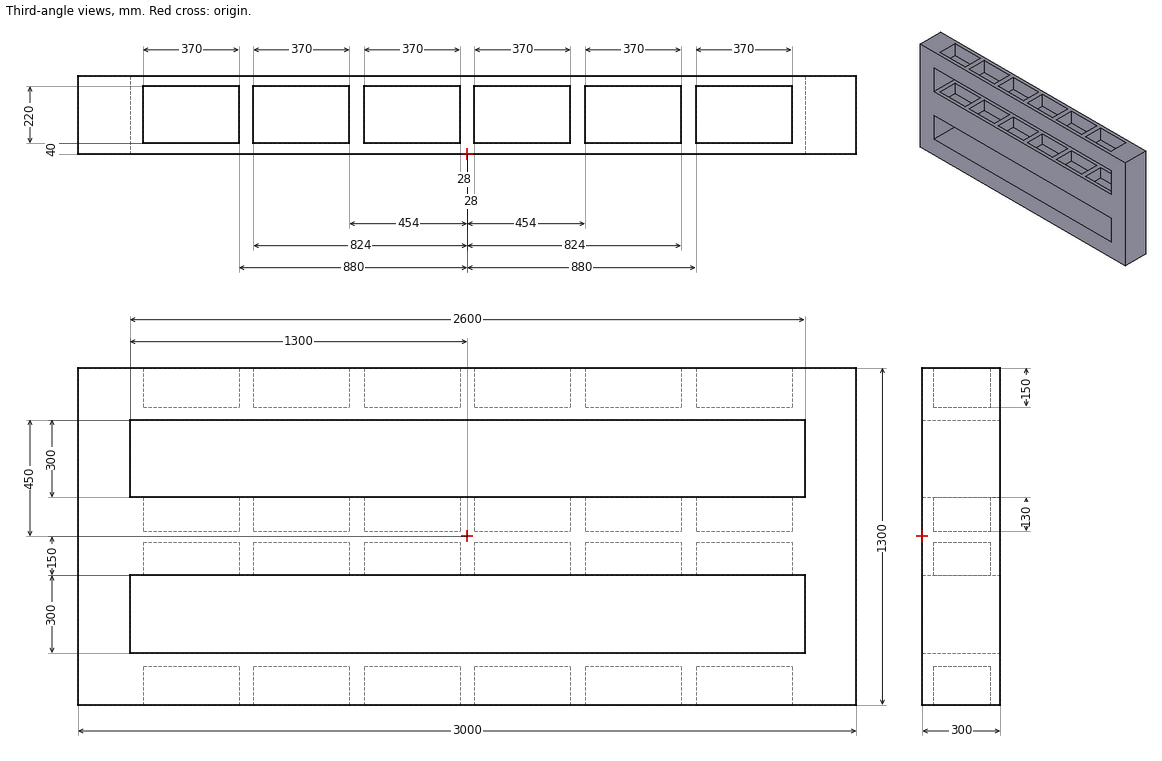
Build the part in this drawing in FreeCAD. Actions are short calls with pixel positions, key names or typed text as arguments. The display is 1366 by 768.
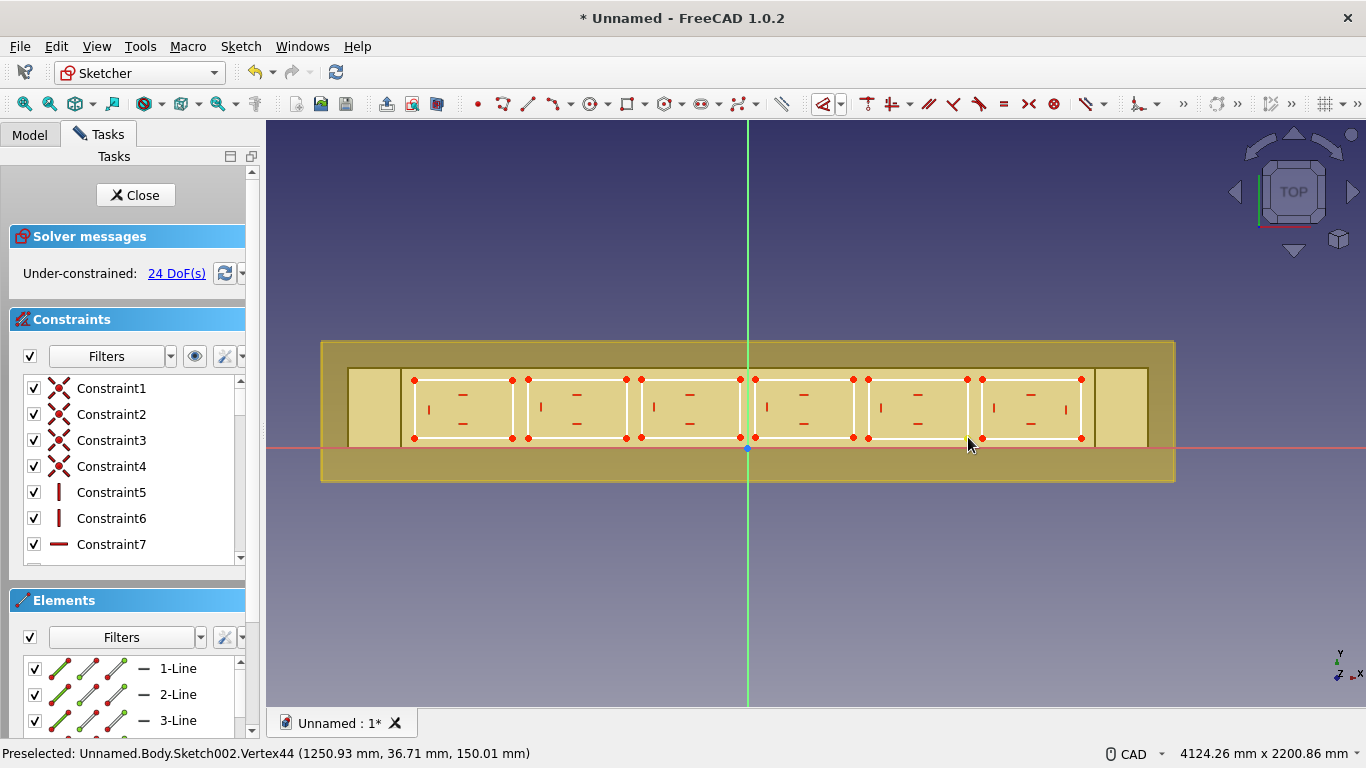
click(415, 398)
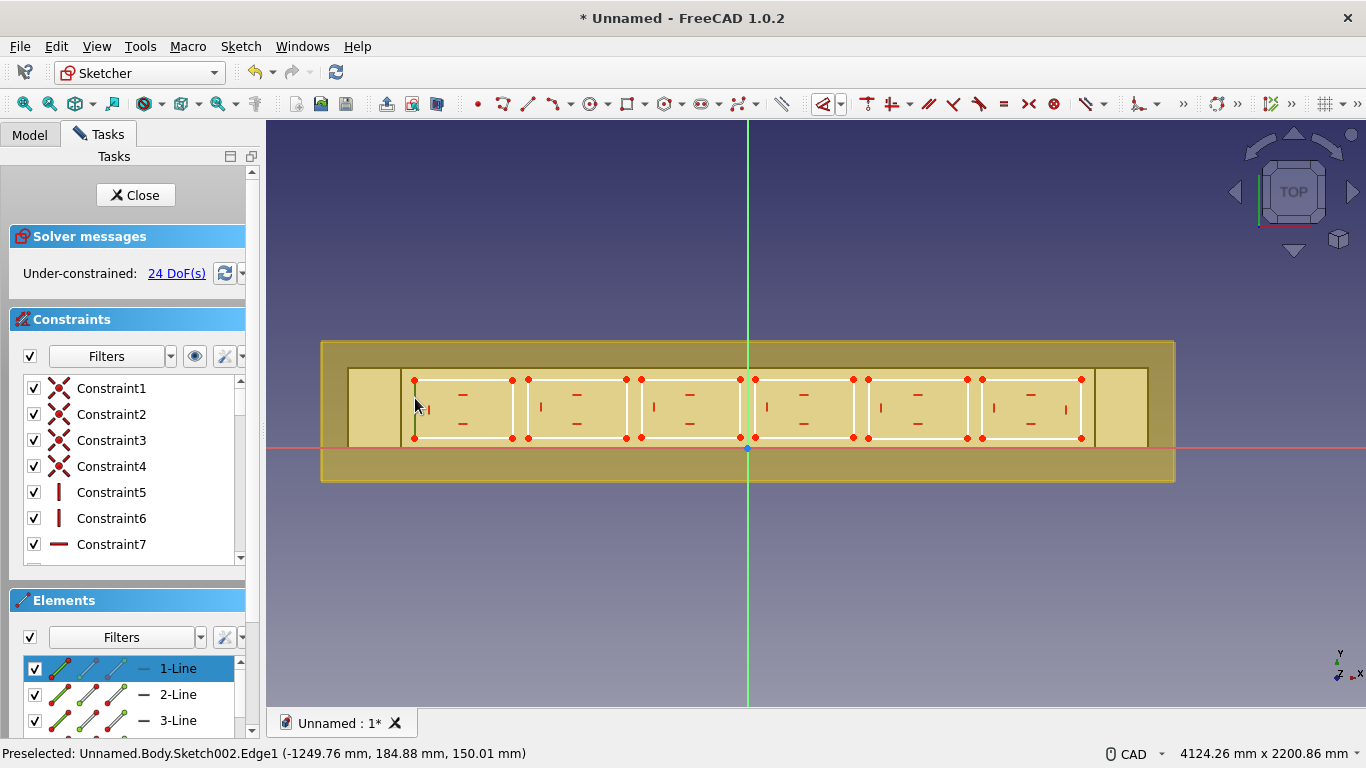
key(i)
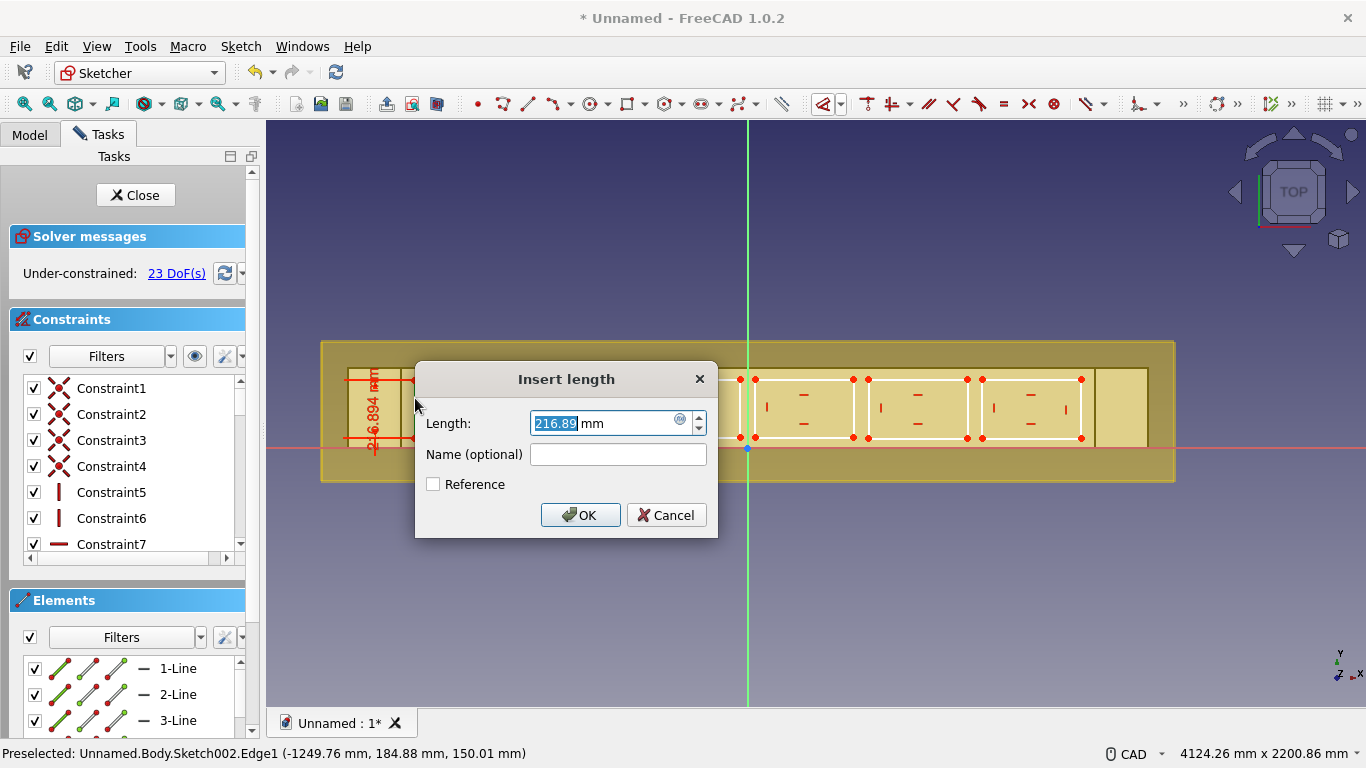
text(220)
key(Return)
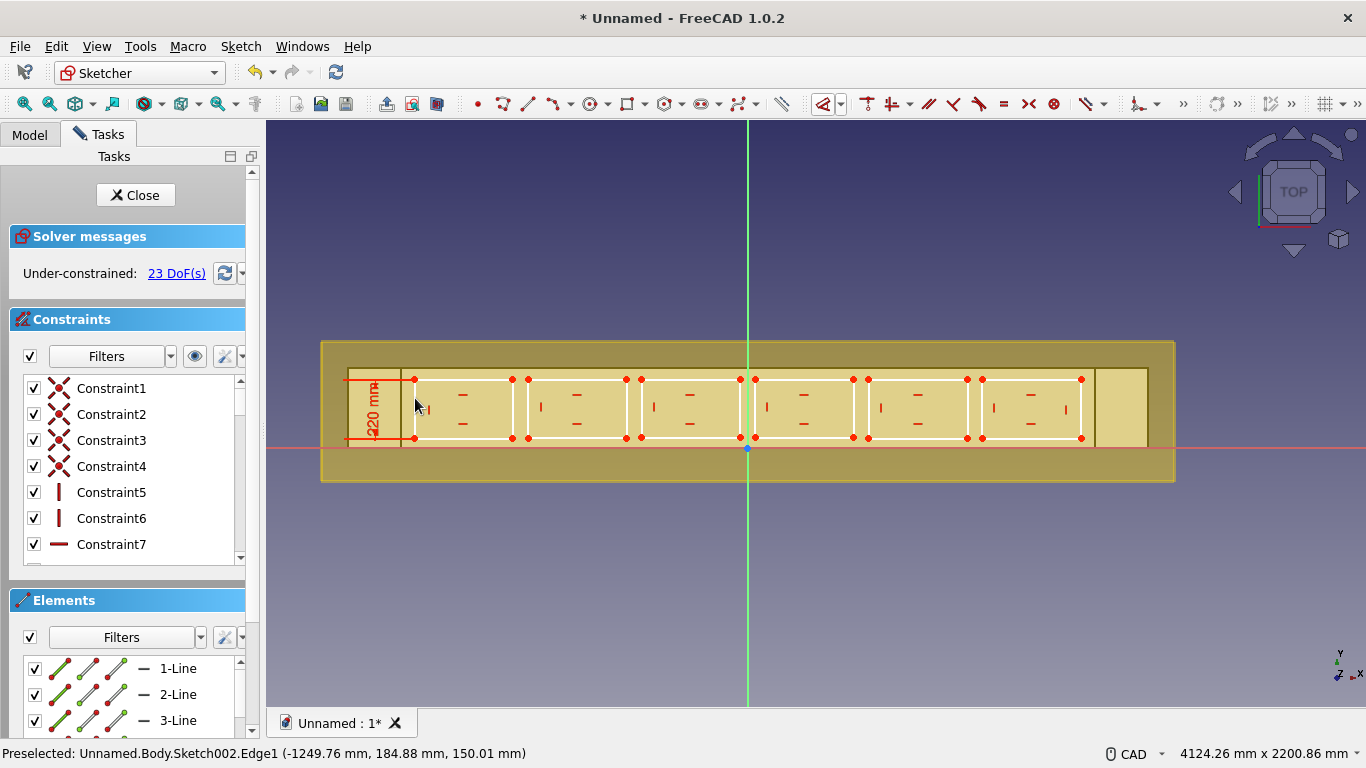
scroll(444, 439, up, 2)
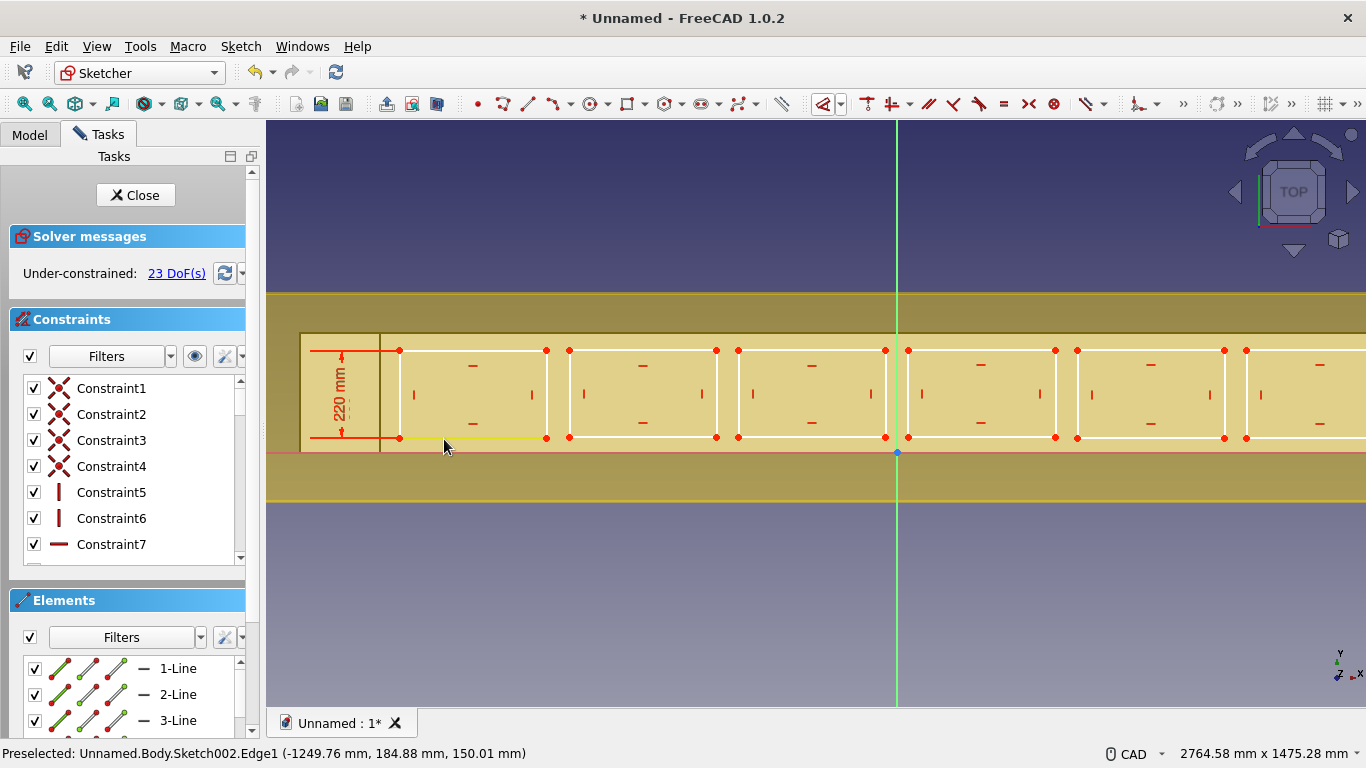
click(444, 438)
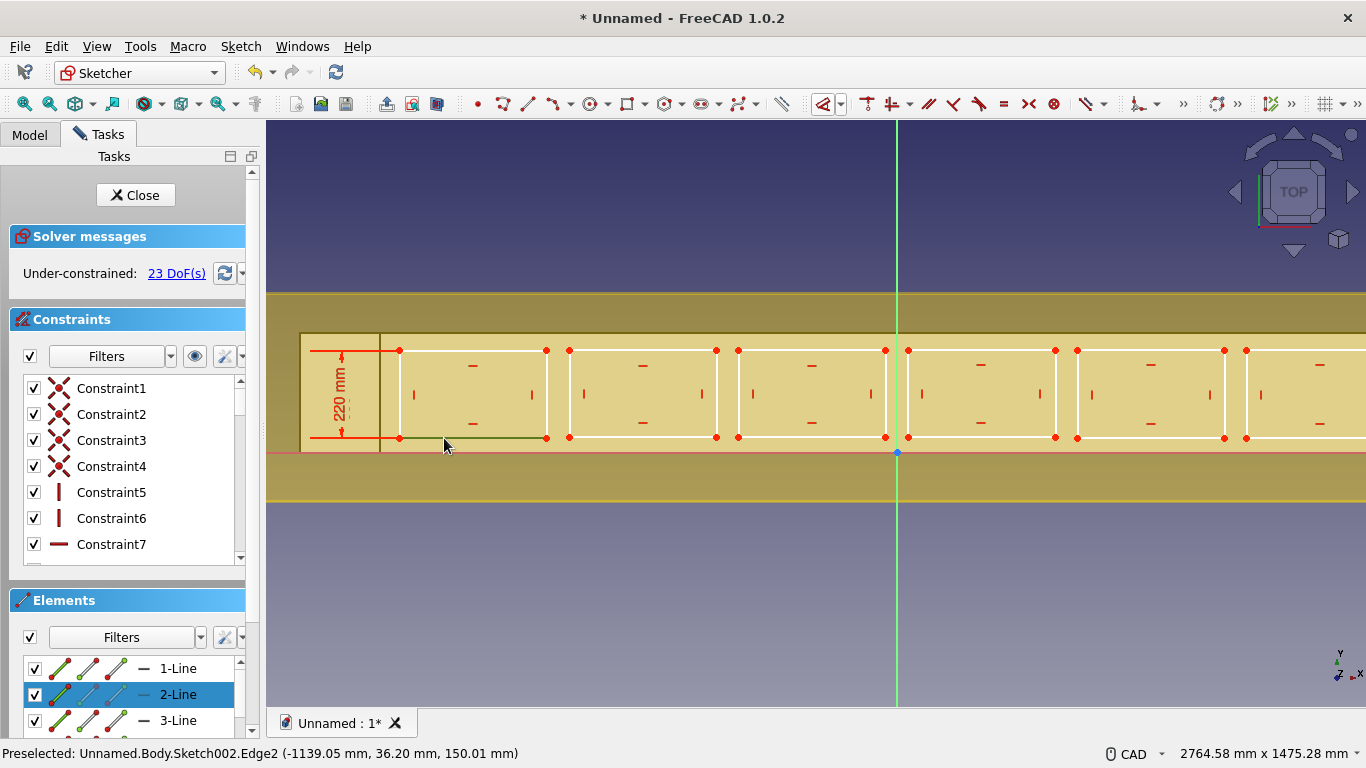
key(l)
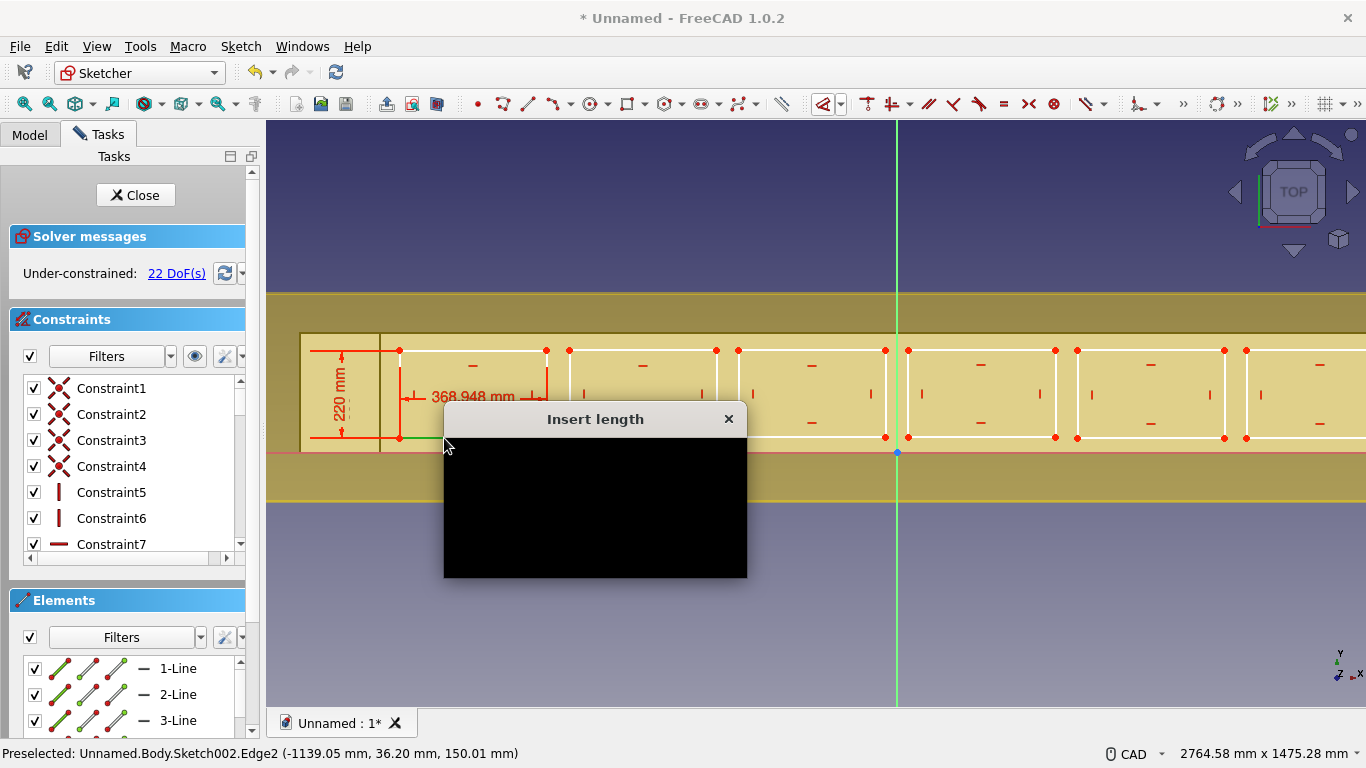
text(370)
key(Return)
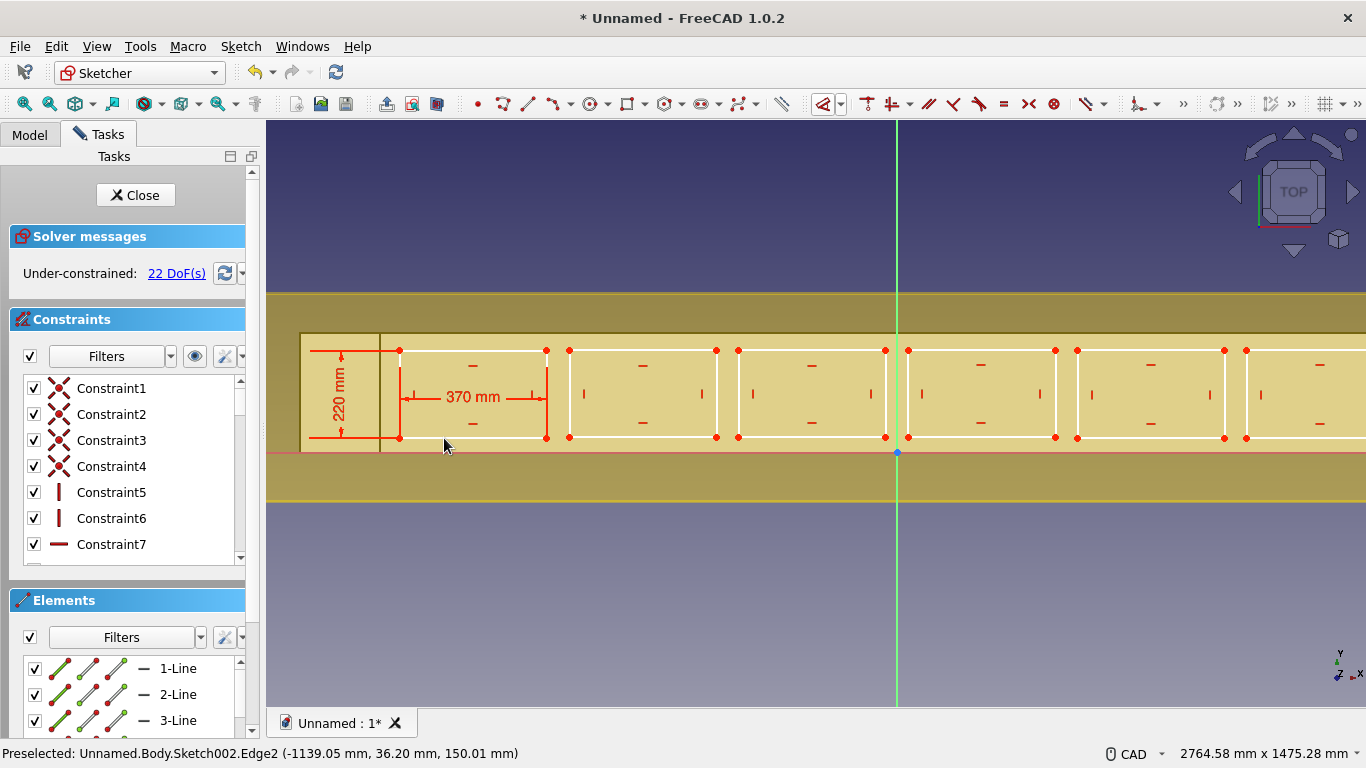
click(570, 376)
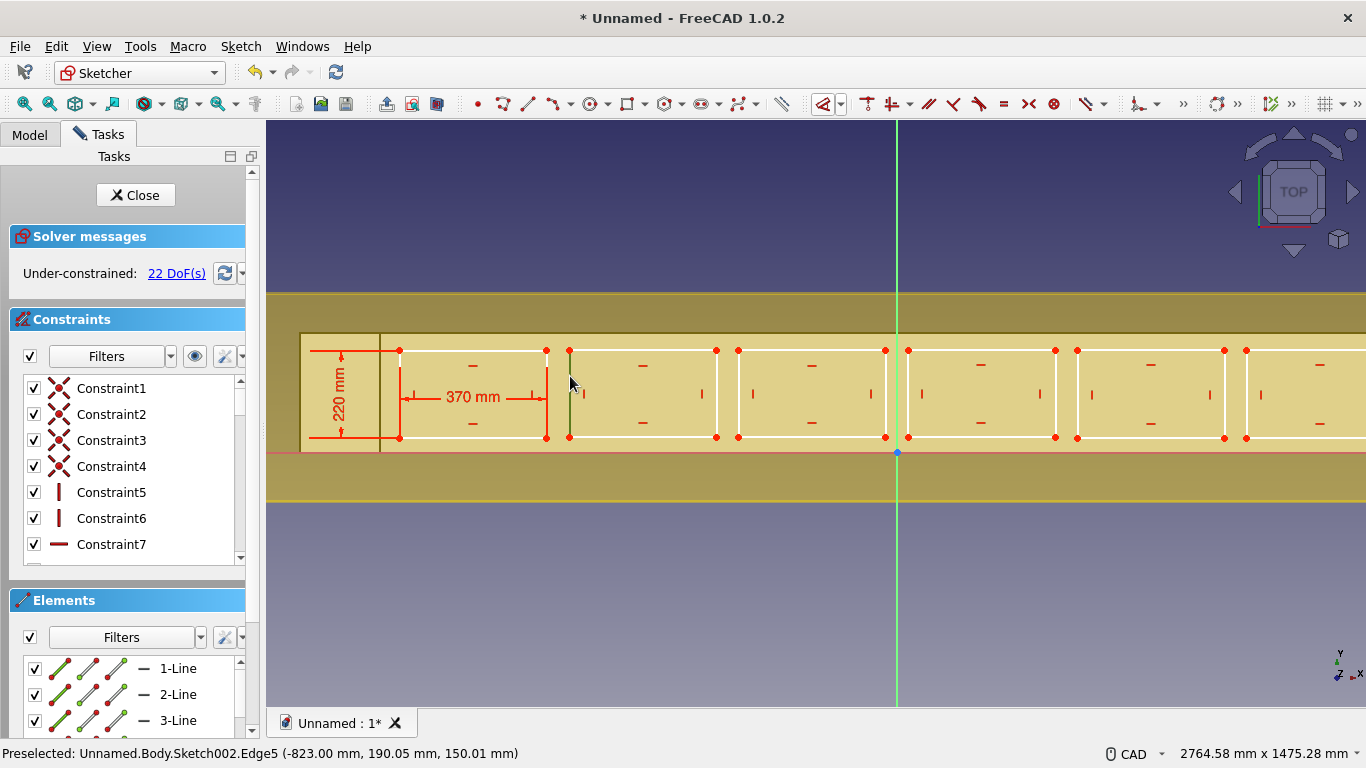
key(i)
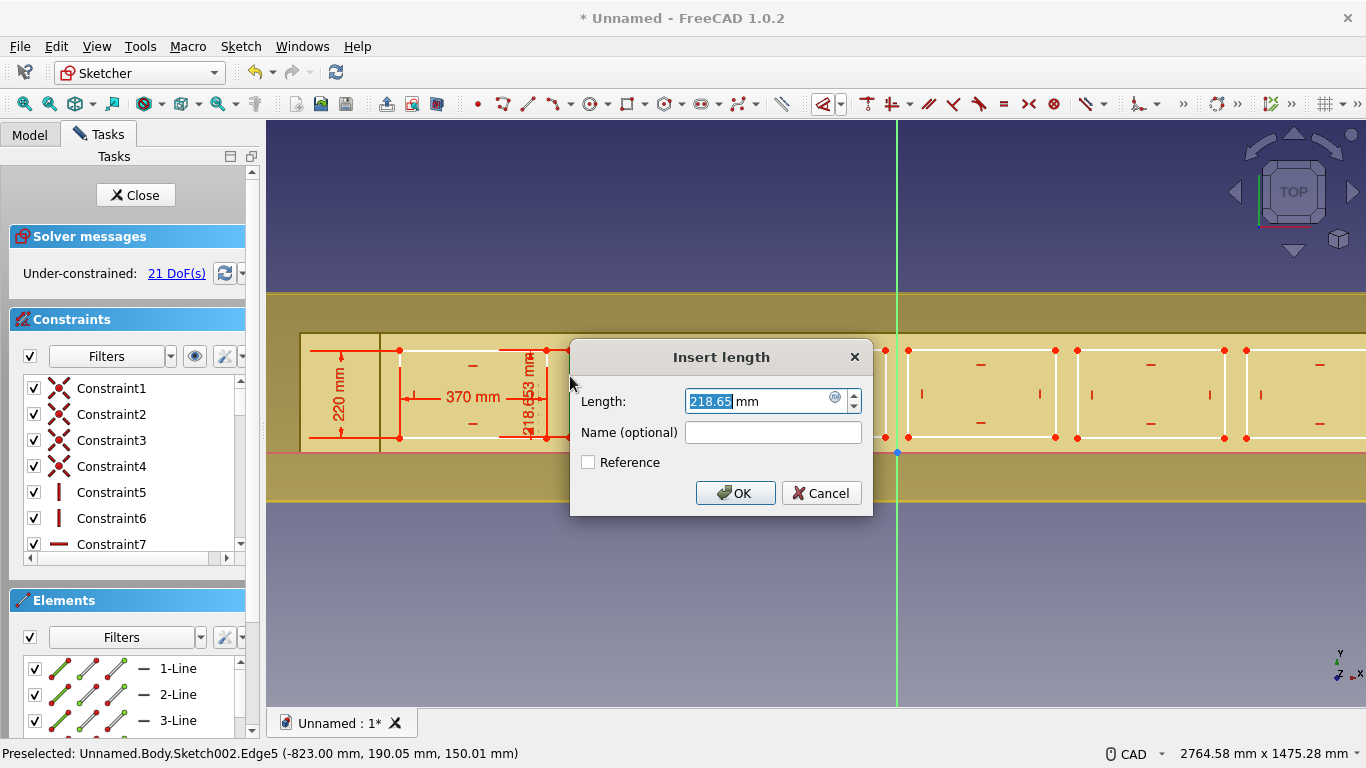
text(220)
key(Return)